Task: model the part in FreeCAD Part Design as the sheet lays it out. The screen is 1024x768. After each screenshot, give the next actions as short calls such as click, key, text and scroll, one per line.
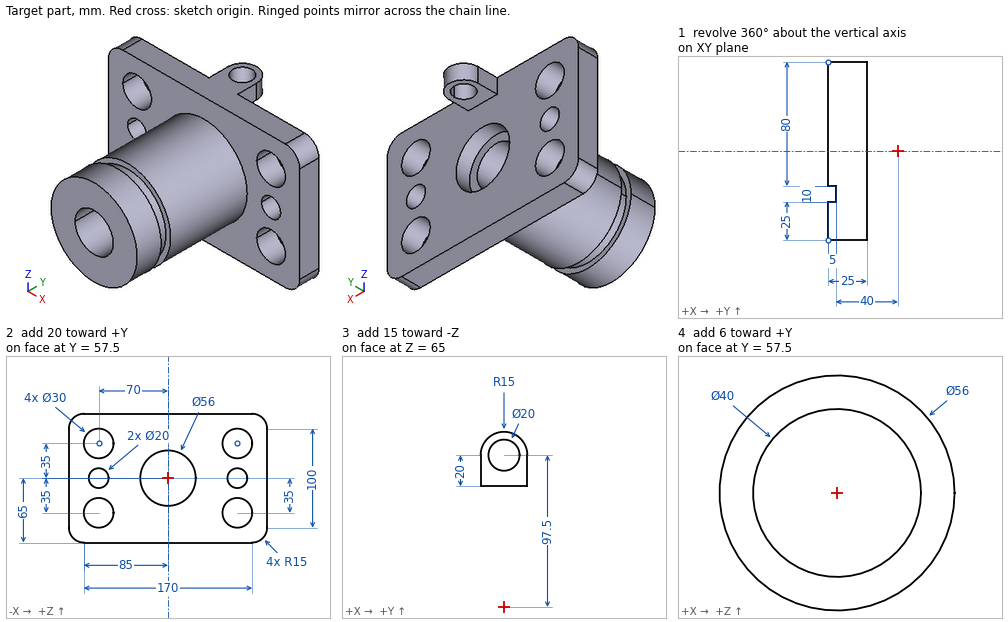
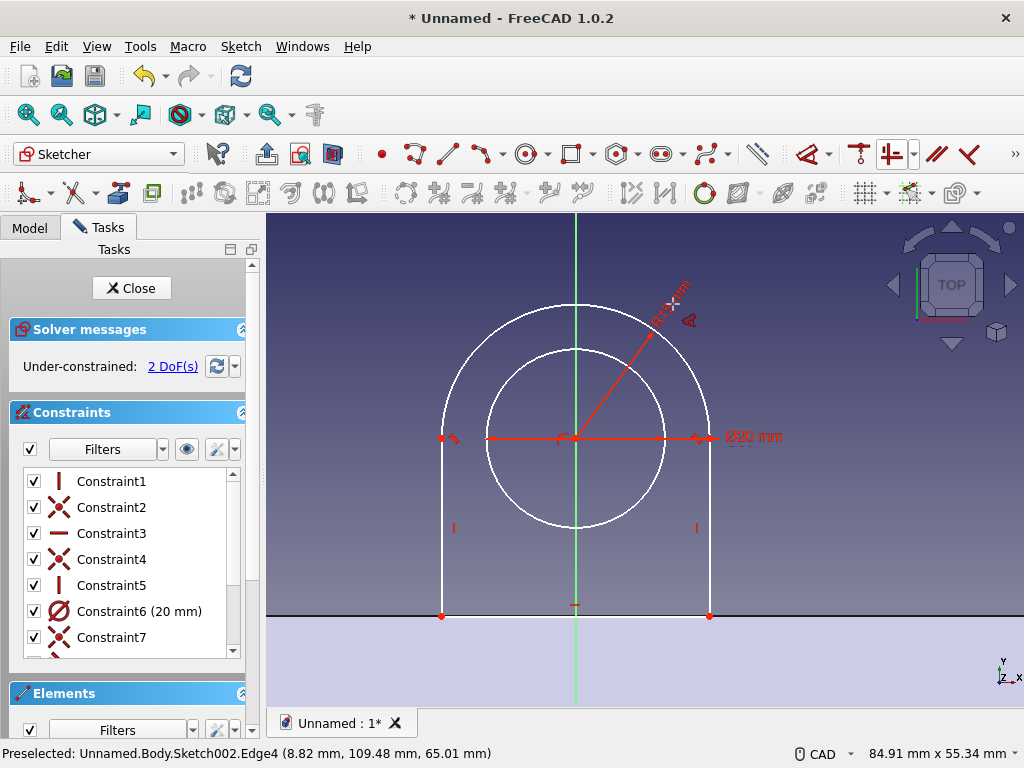
click(442, 492)
click(408, 528)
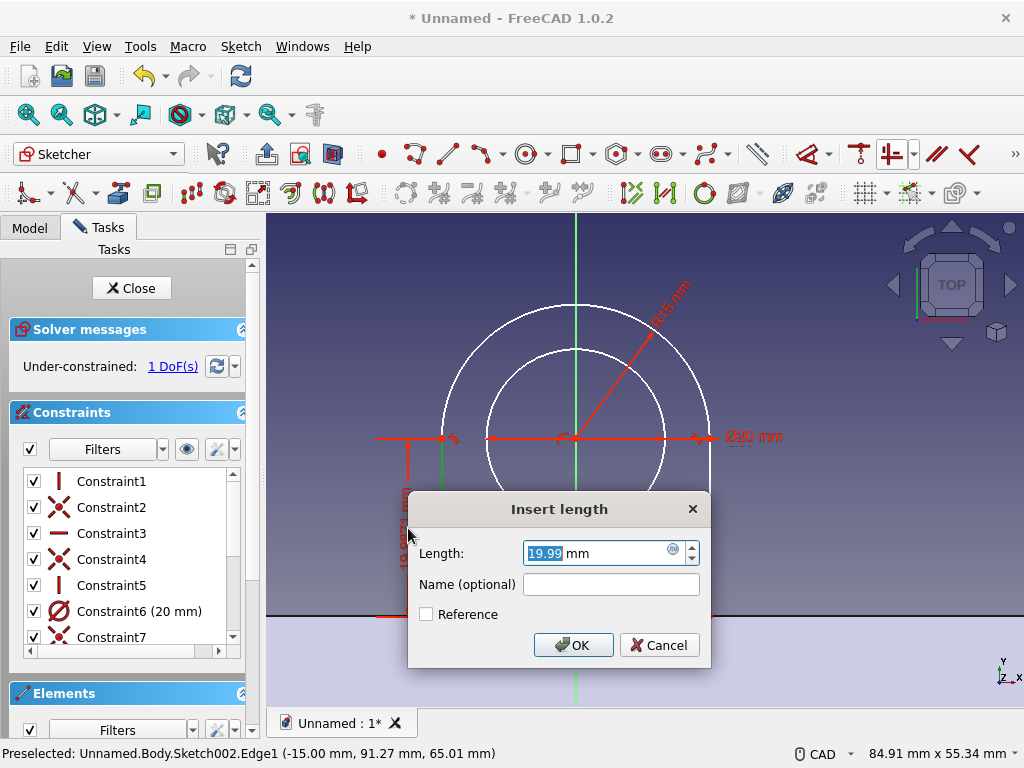
text(20)
key(Return)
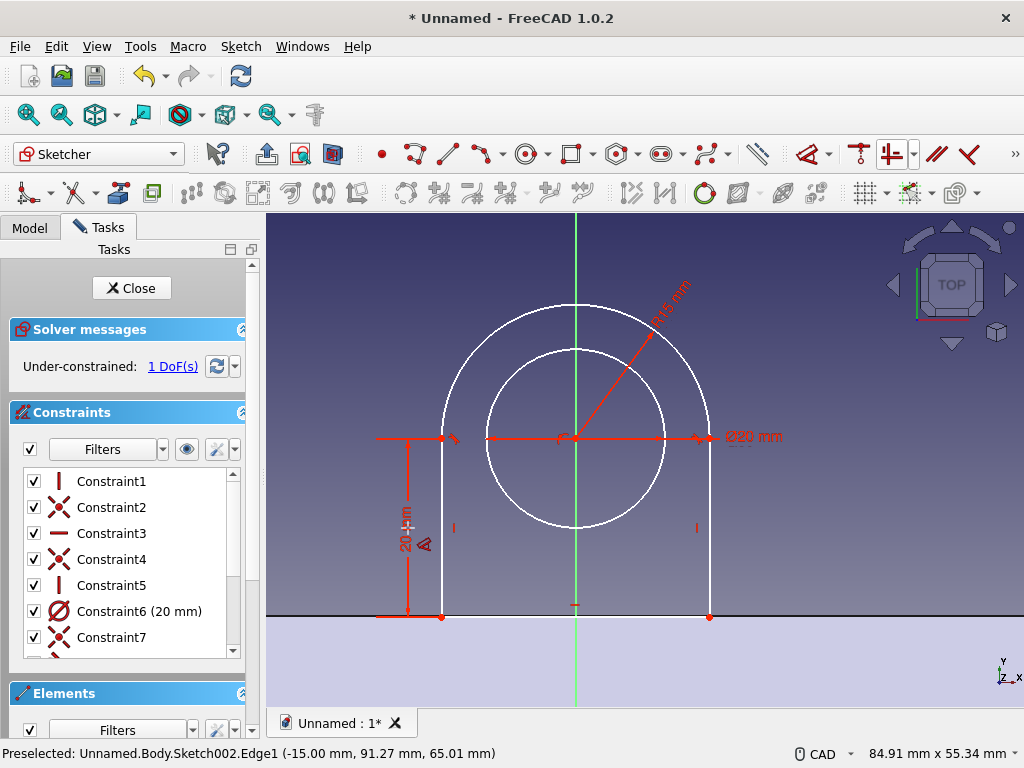
click(576, 439)
click(610, 559)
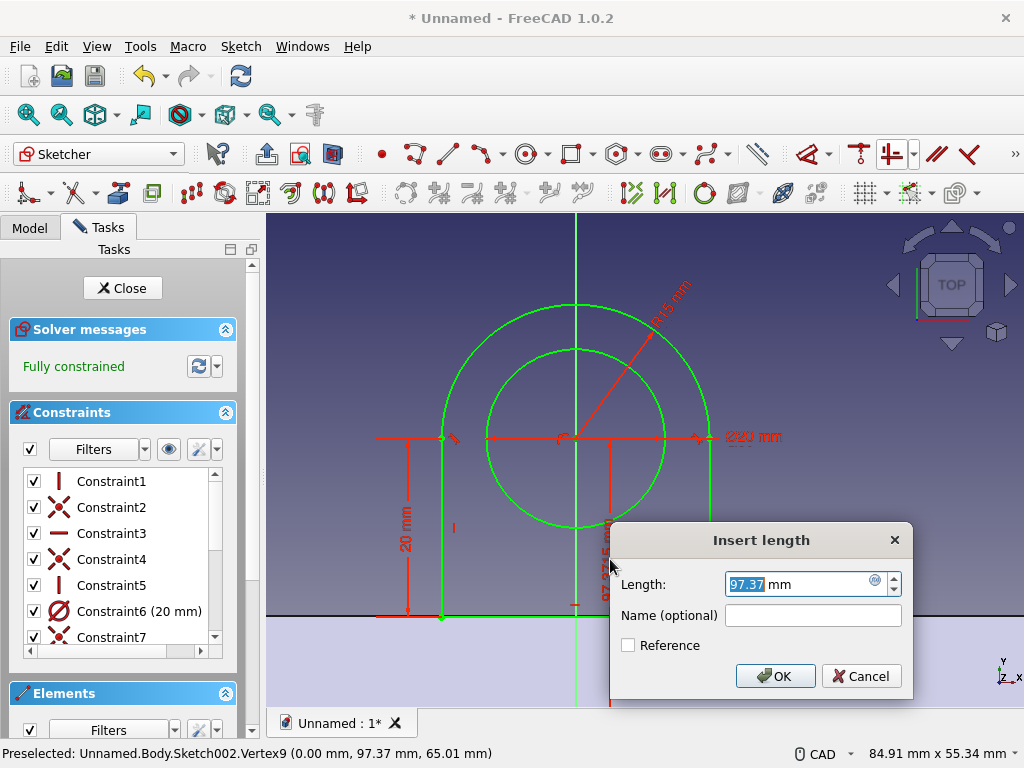
text(97.5)
key(Return)
key(Escape)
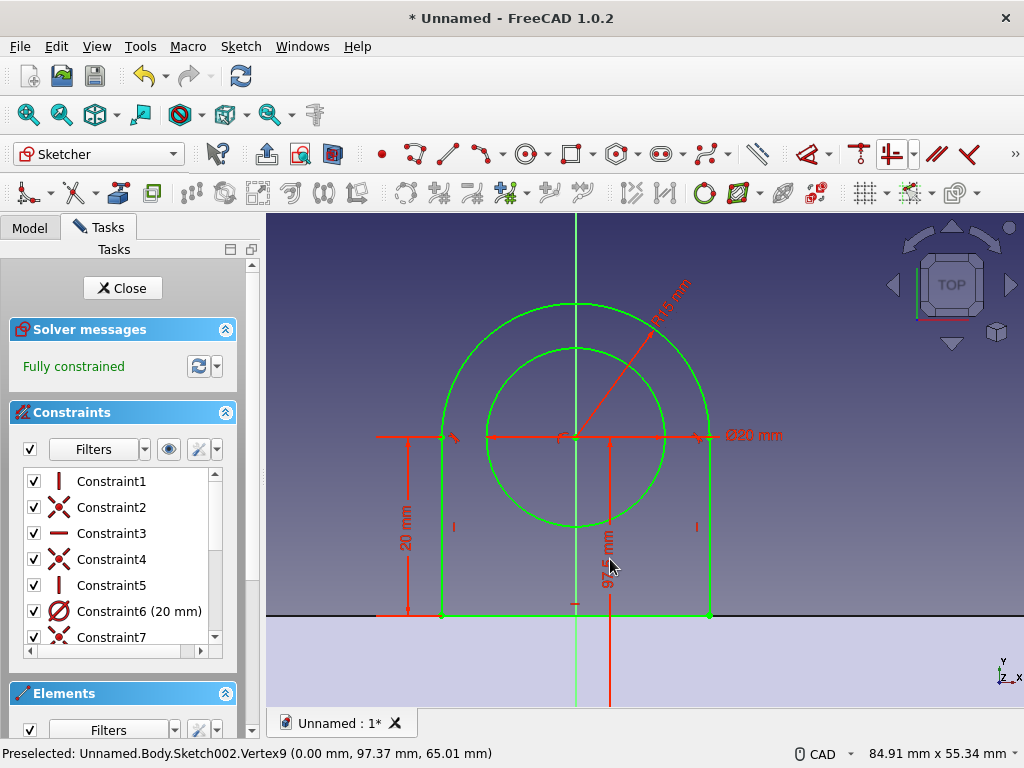
click(123, 288)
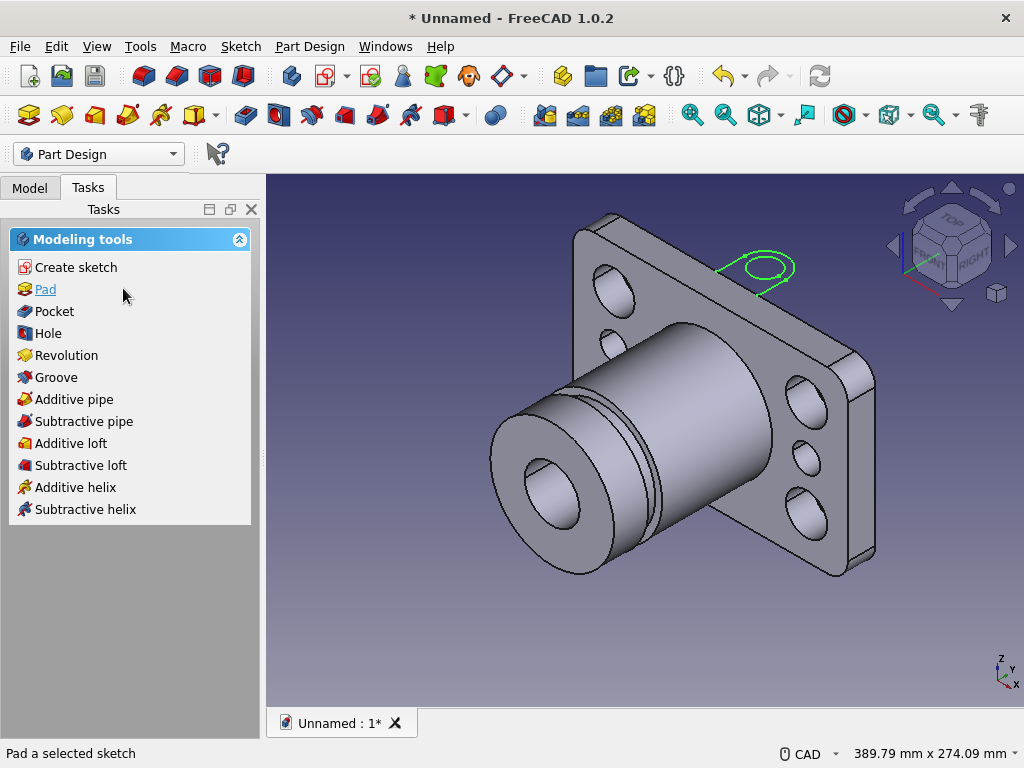
click(29, 116)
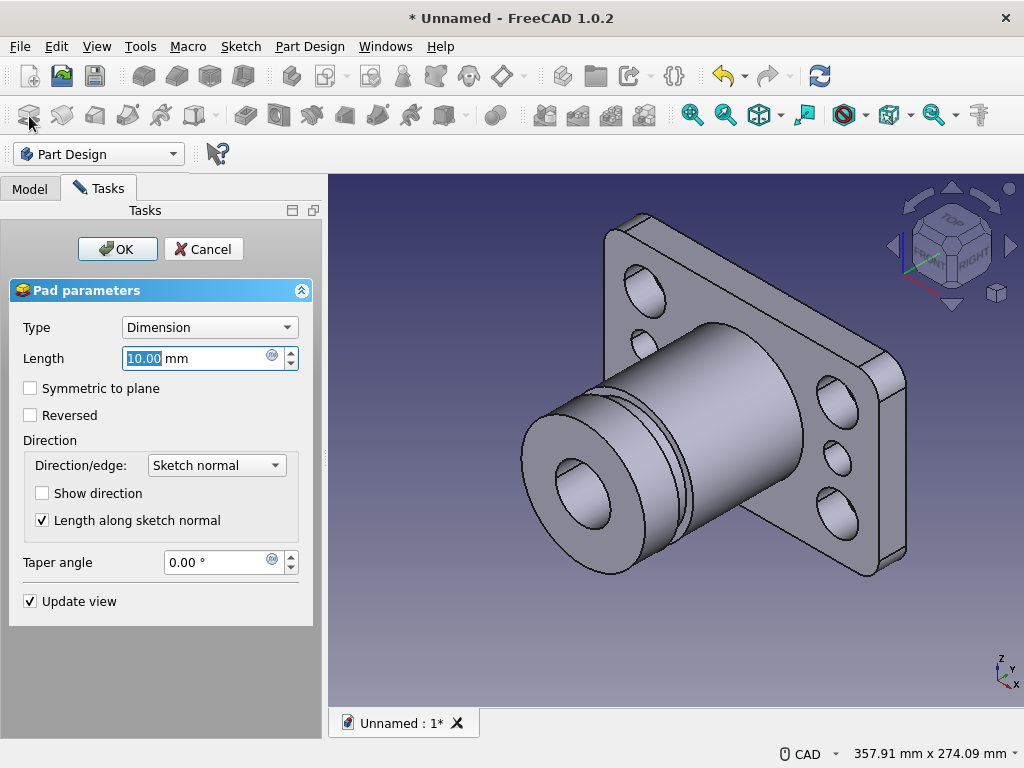
text(15)
key(Tab)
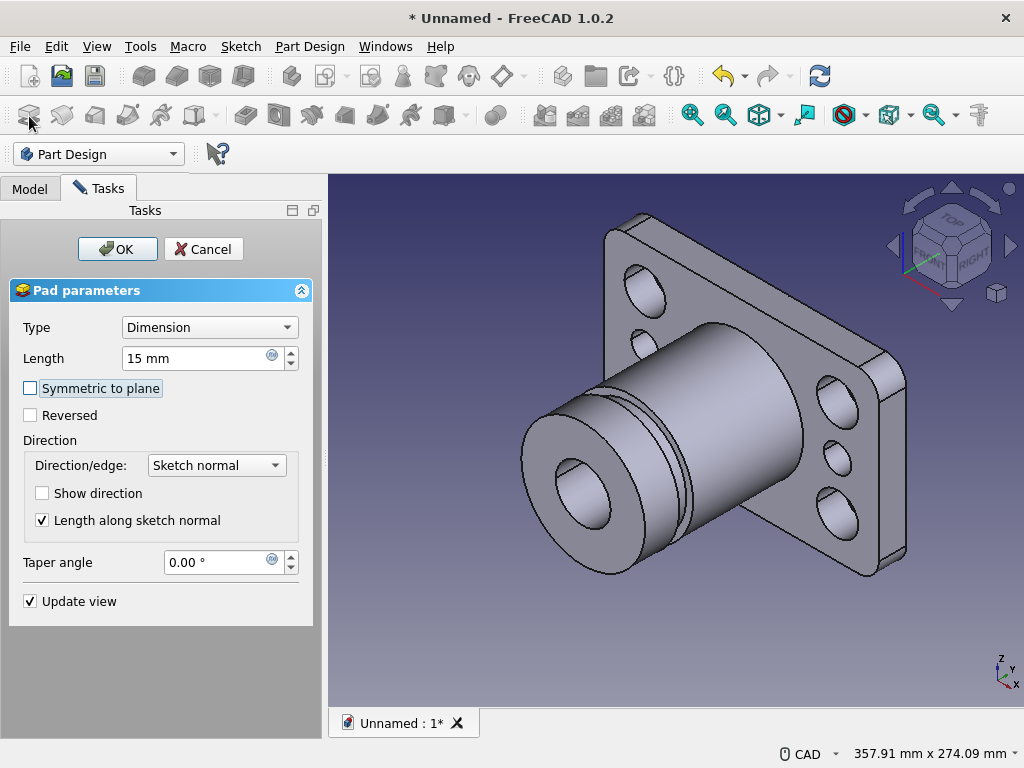
click(31, 415)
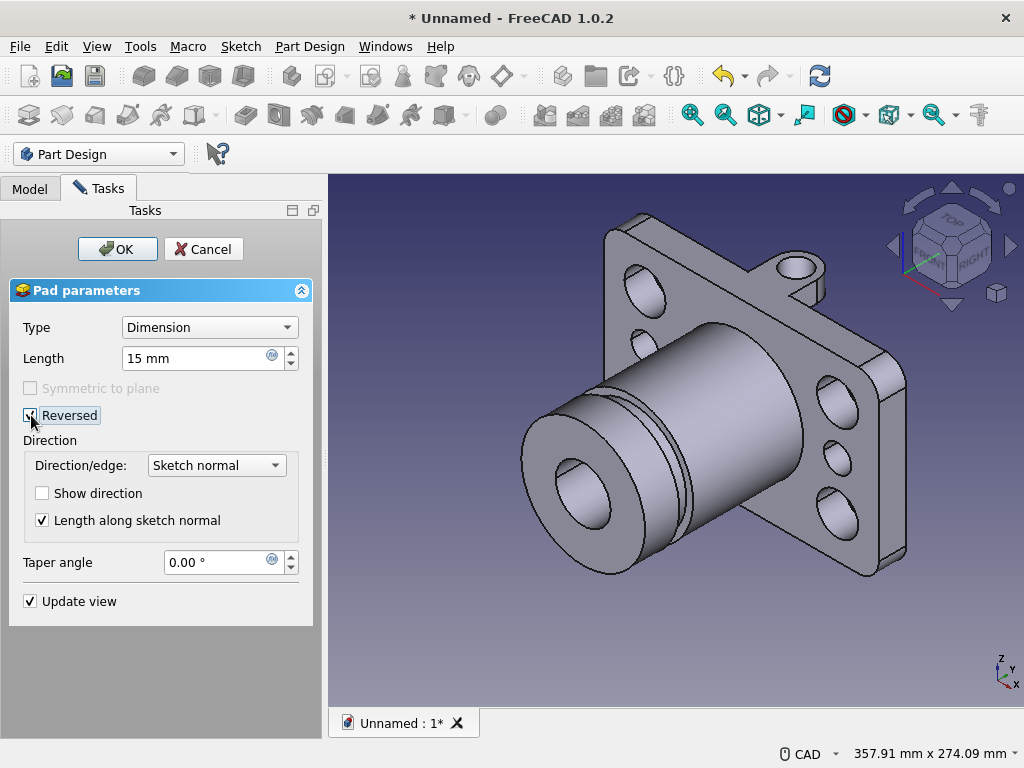
click(118, 249)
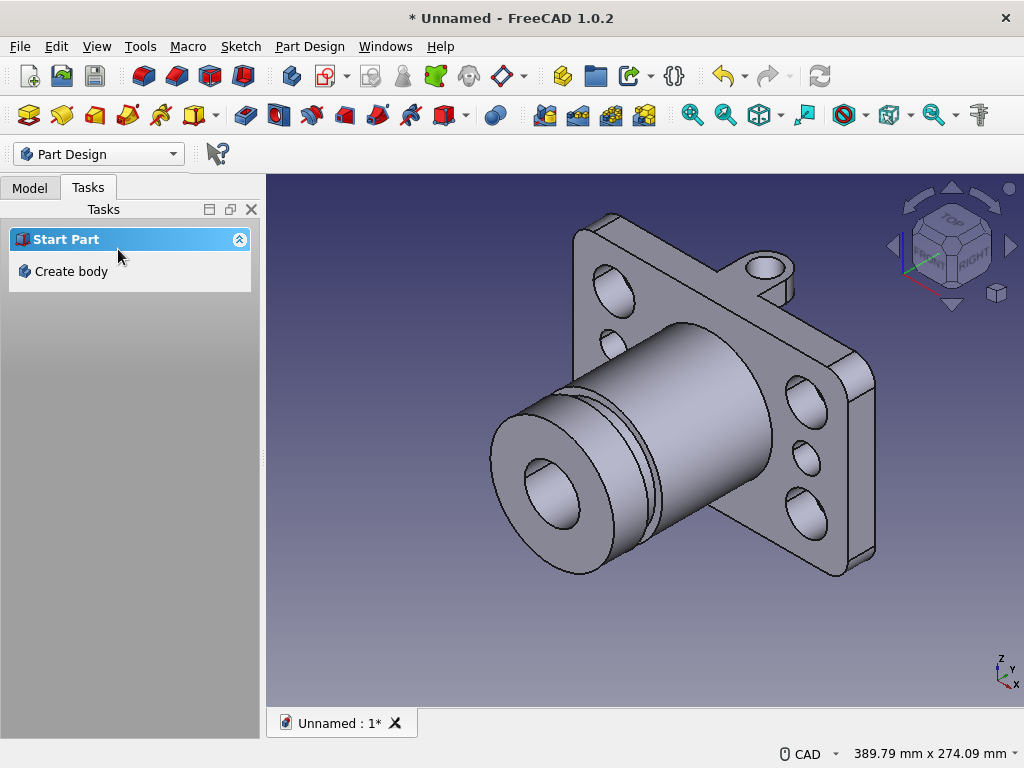
click(789, 359)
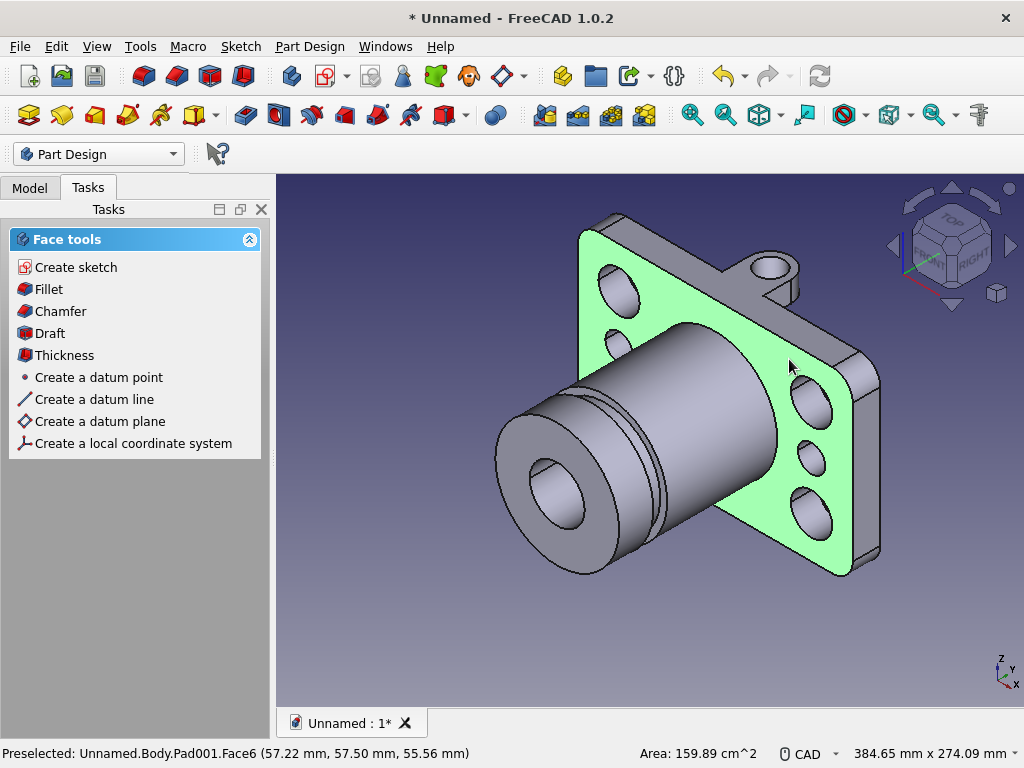
click(324, 76)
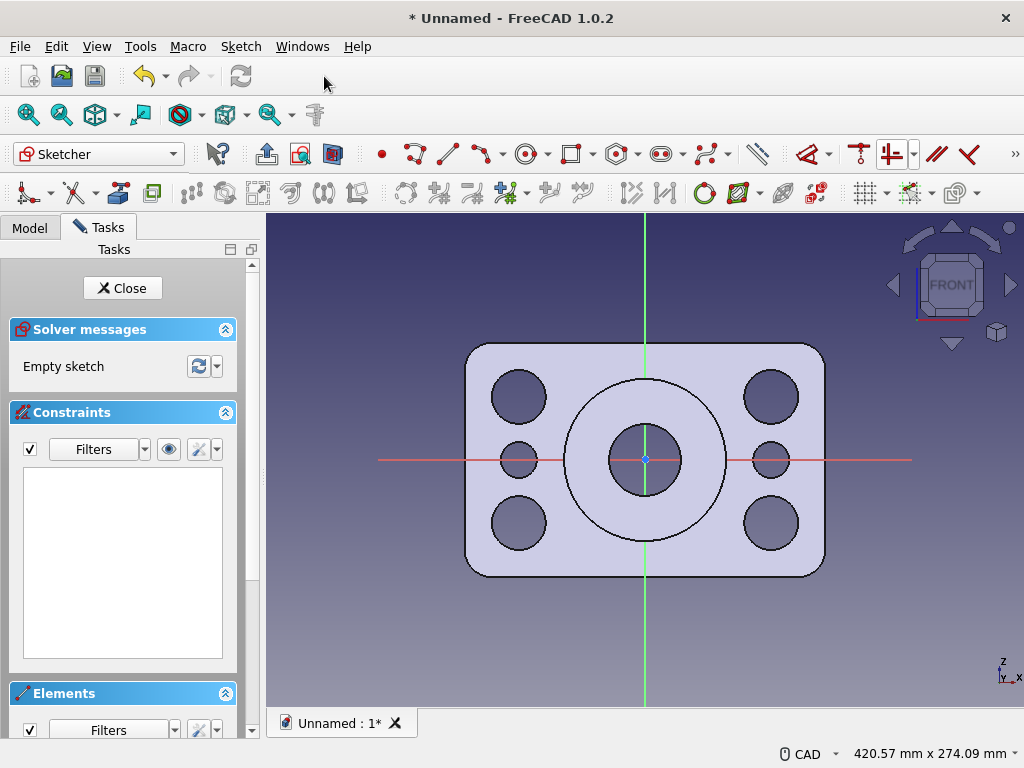
click(333, 154)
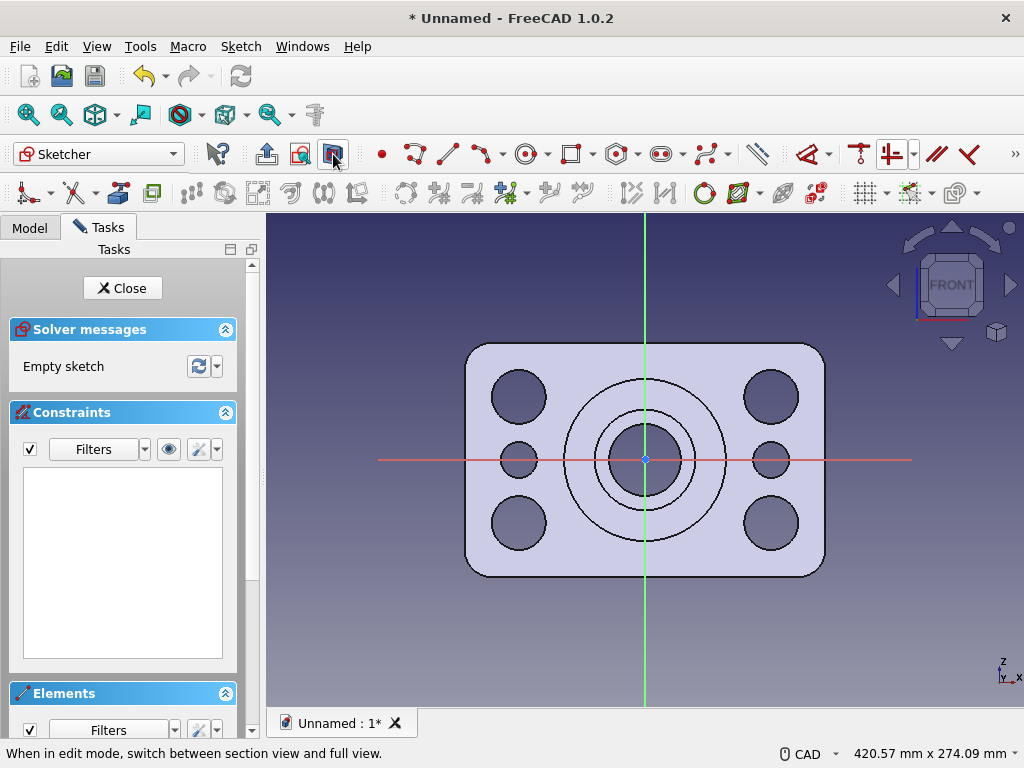
scroll(675, 460, up, 6)